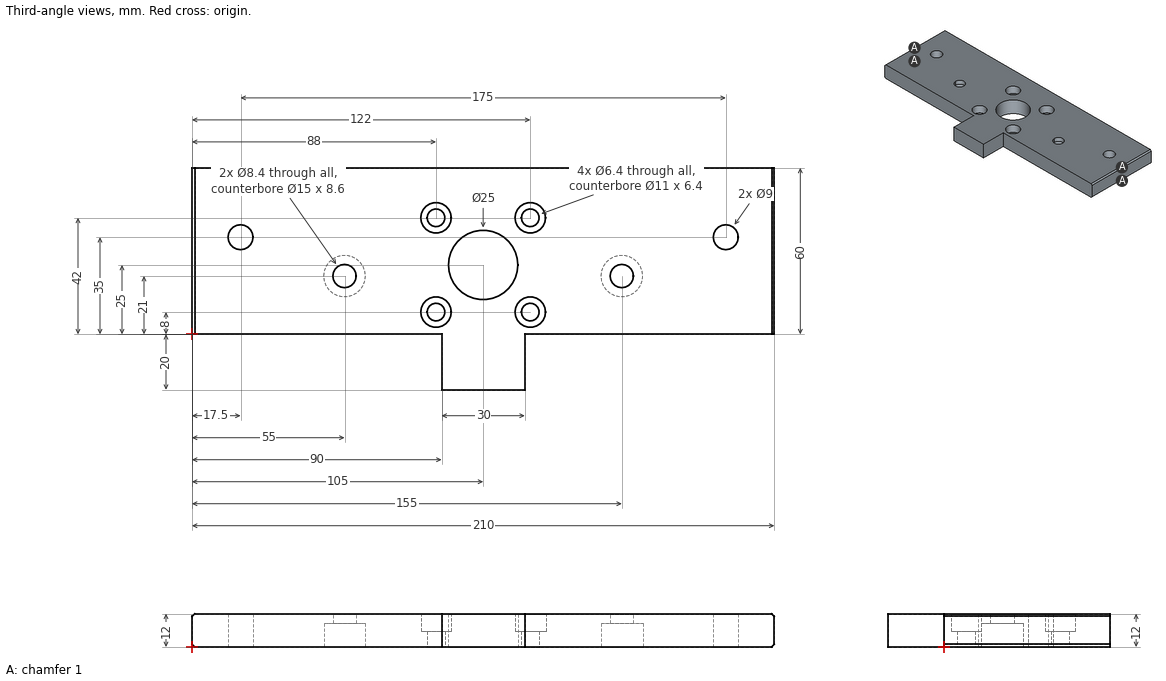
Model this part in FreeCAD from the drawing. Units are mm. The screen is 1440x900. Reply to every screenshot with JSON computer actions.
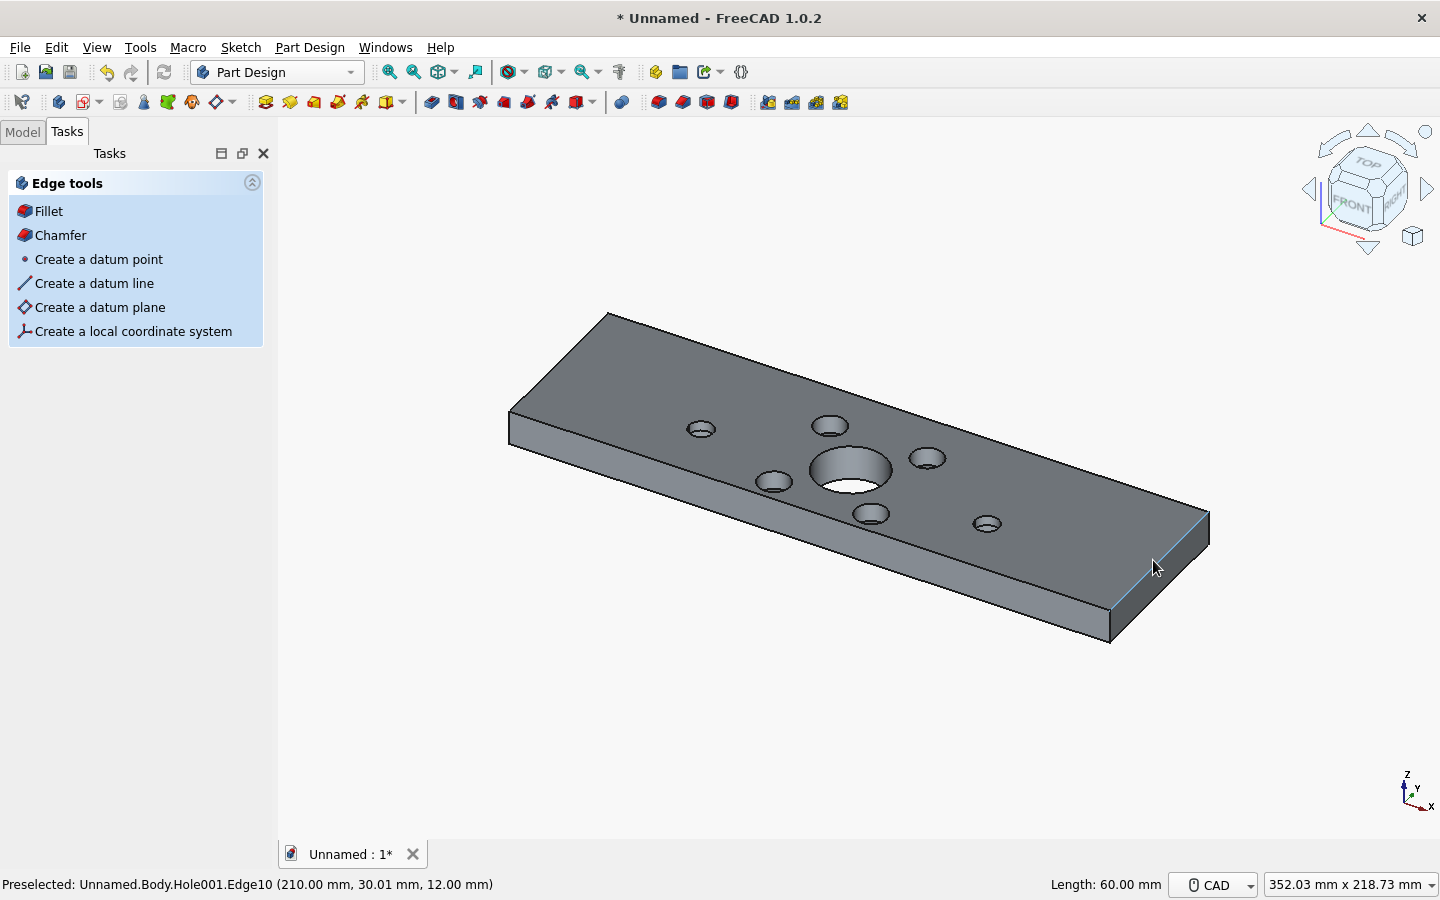
{"action": "key", "text": "0"}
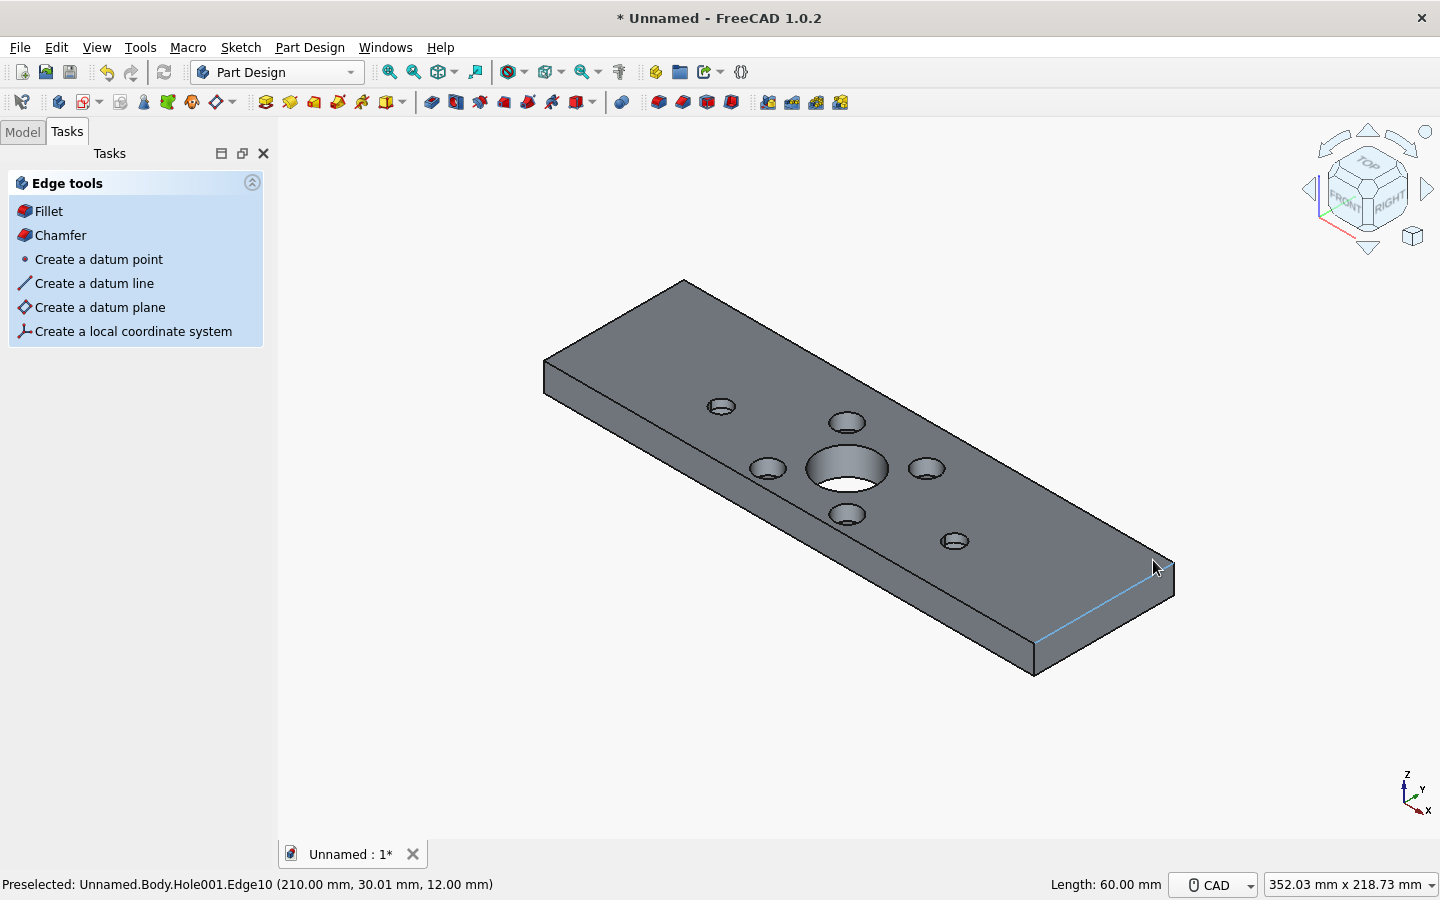
{"action": "key", "text": "2"}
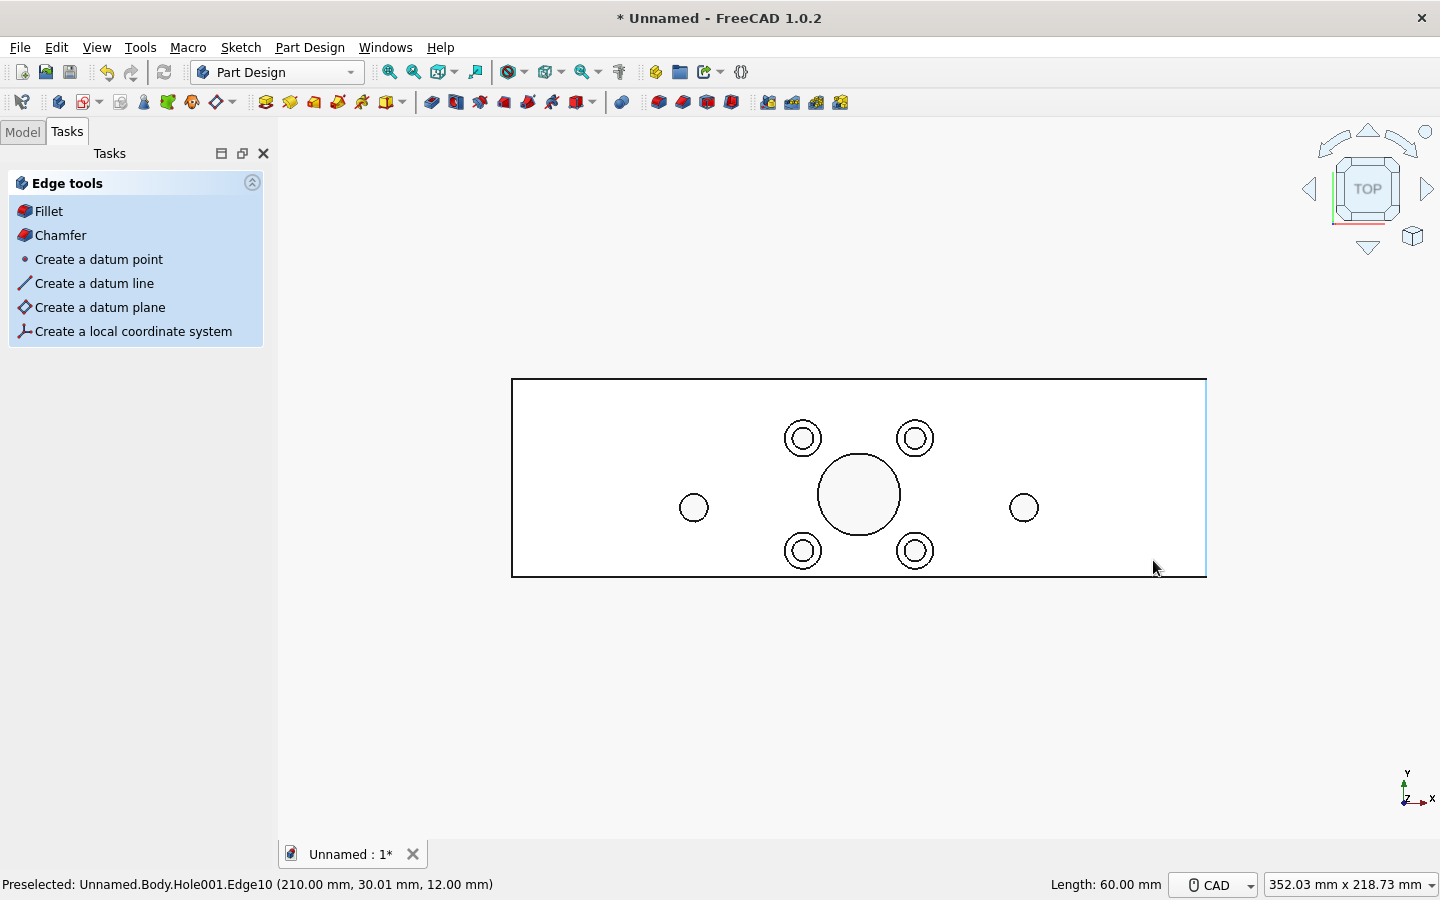
{"action": "left_click", "coordinate": [512, 477], "text": "ctrl"}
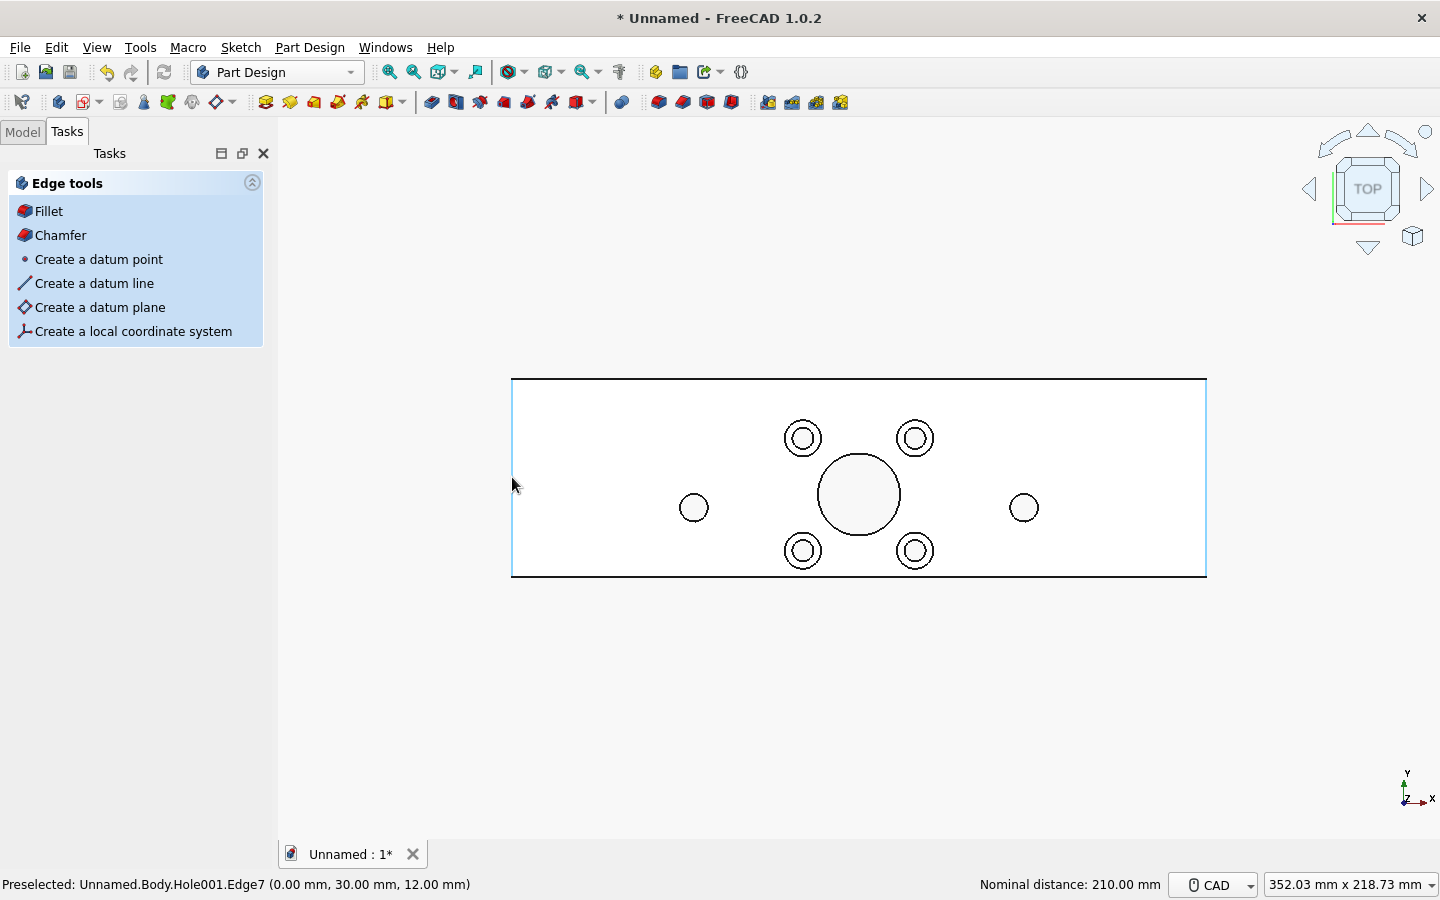
{"action": "key", "text": "1"}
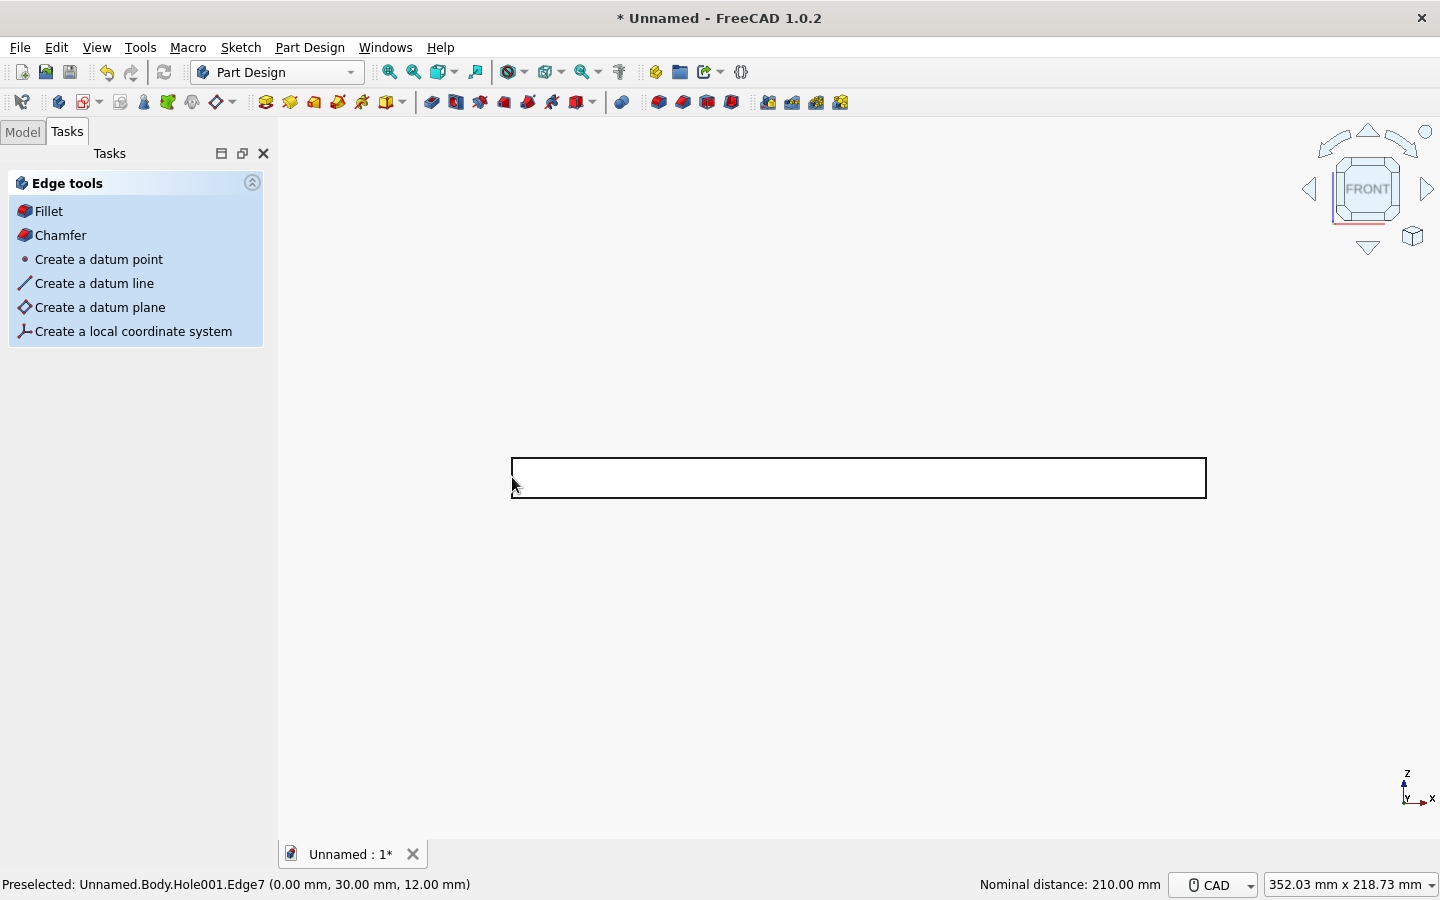
{"action": "key", "text": "3"}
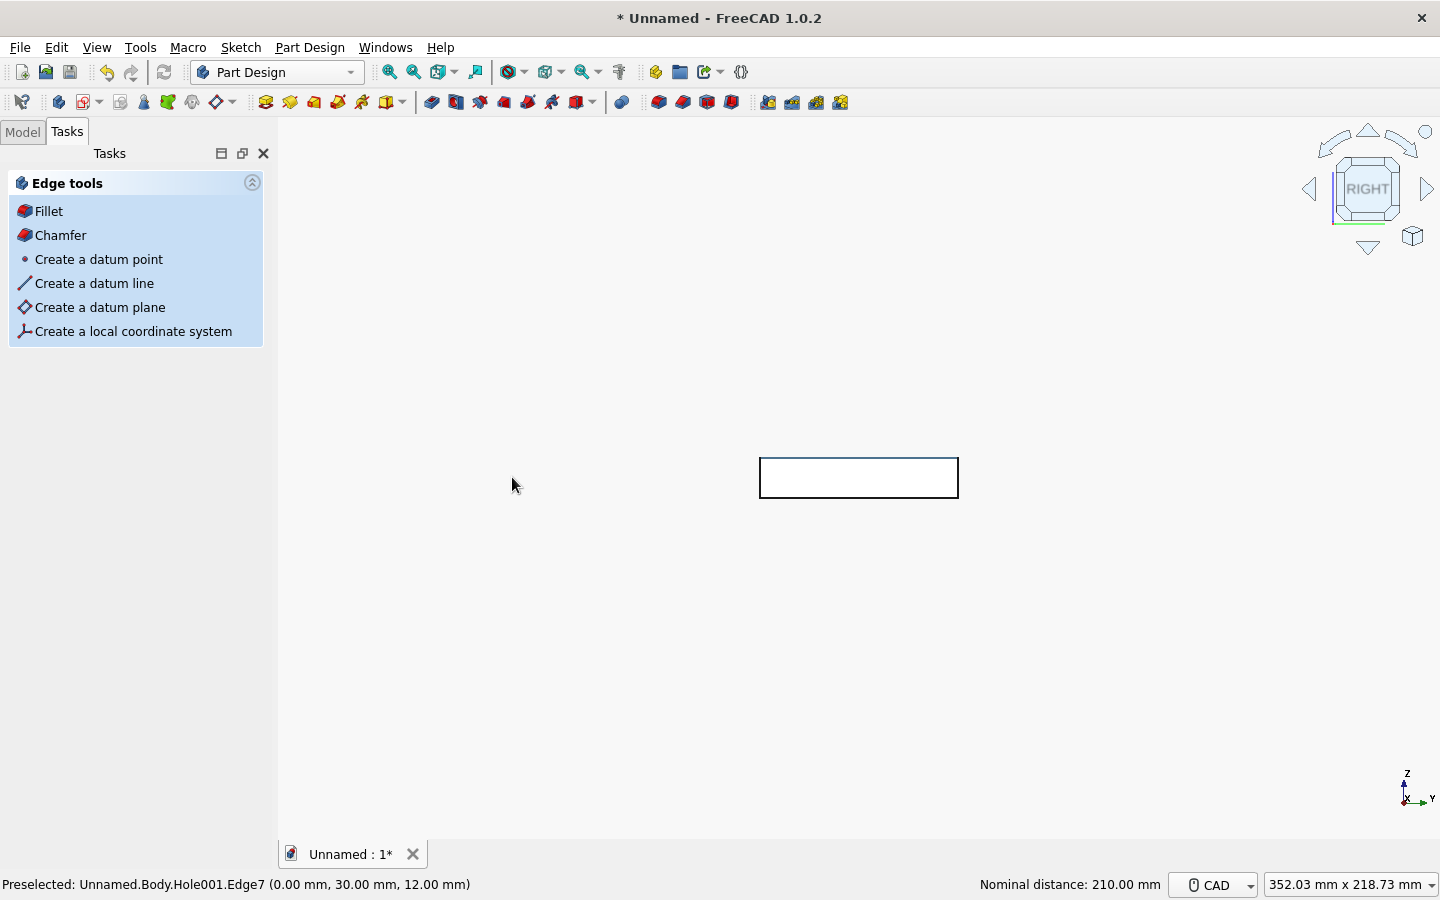
{"action": "key", "text": "v f"}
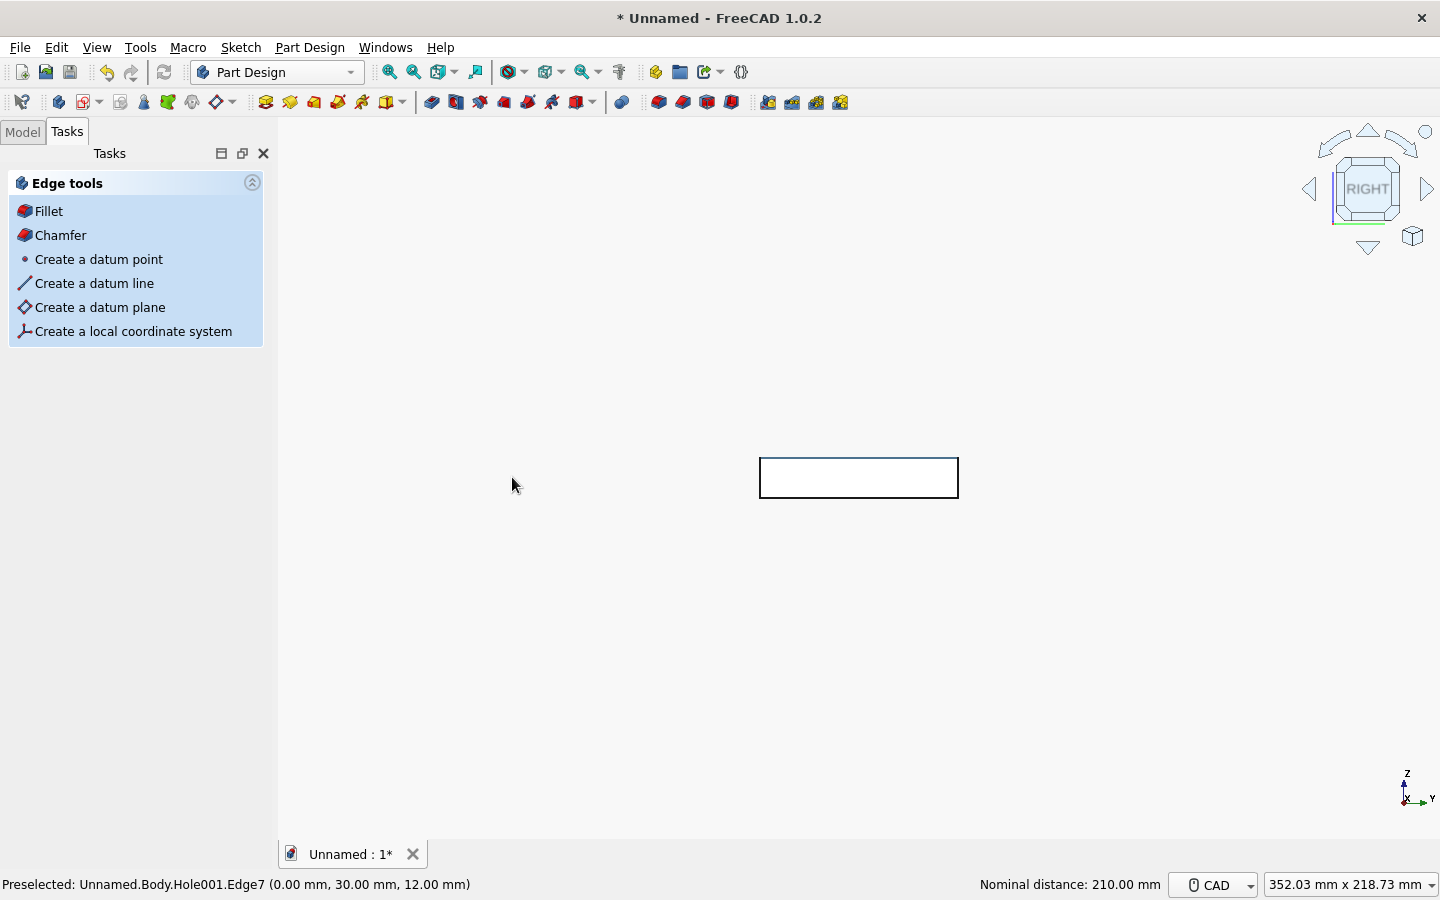
{"action": "left_click", "coordinate": [859, 497], "text": "ctrl"}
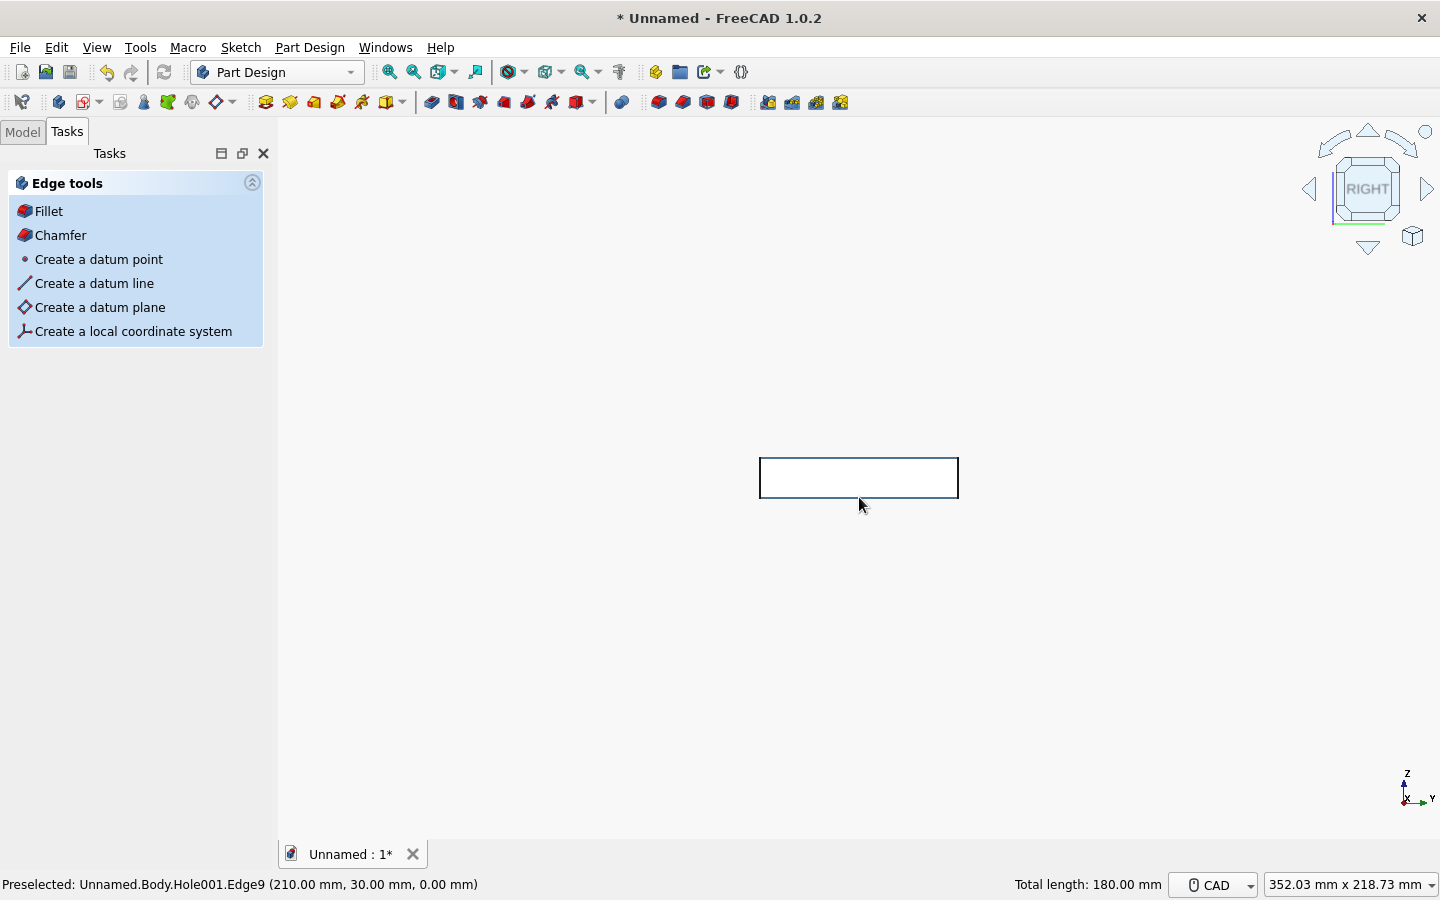
{"action": "key", "text": "5"}